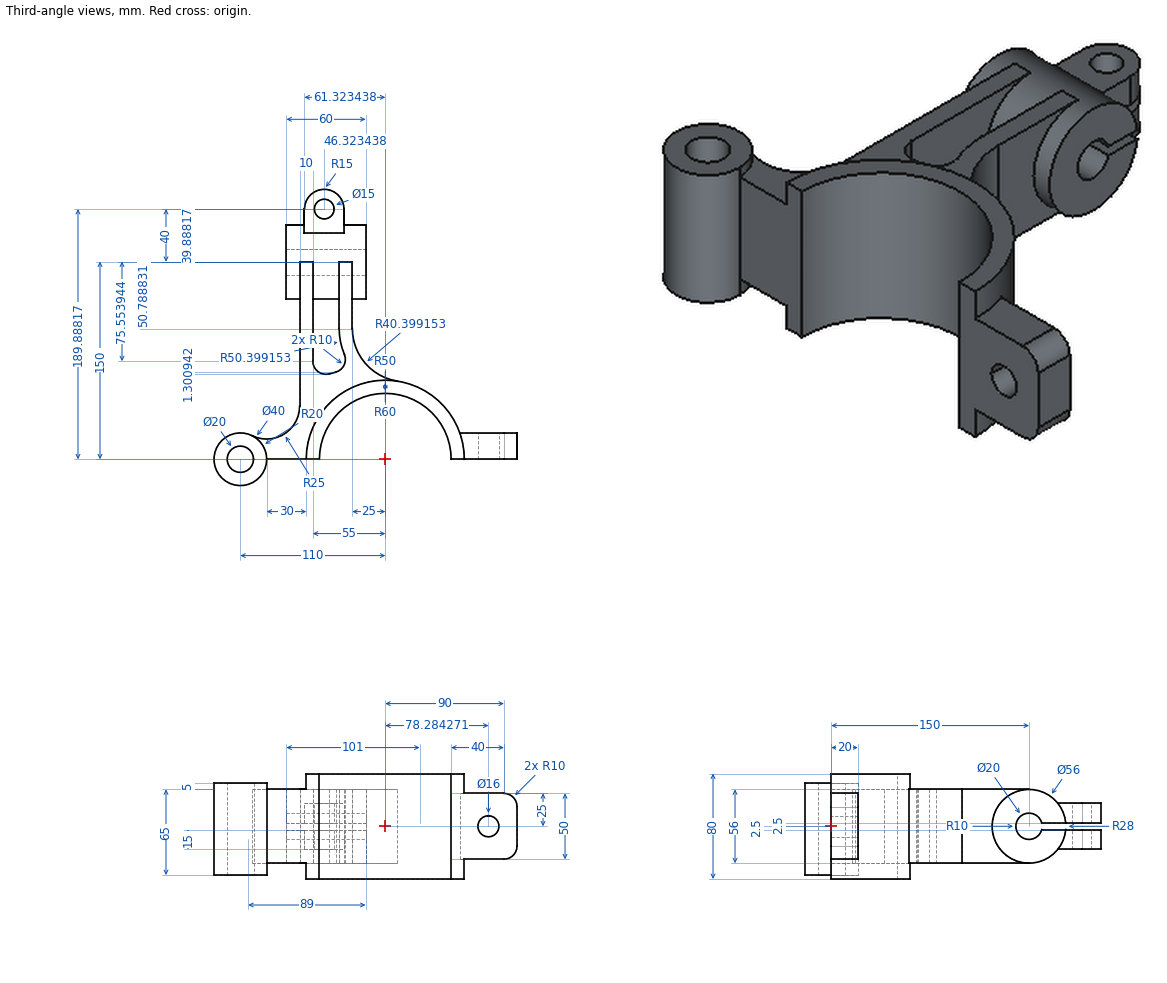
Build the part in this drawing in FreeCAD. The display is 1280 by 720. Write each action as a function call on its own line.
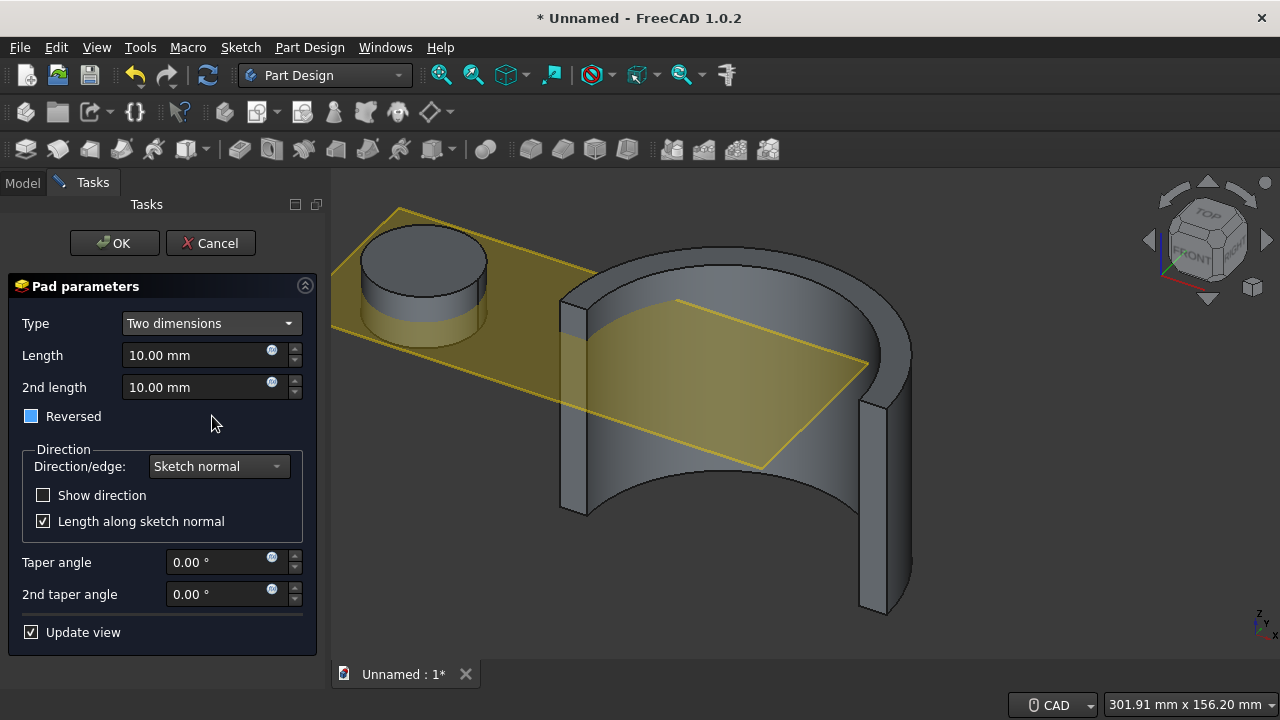
triple_click(204, 355)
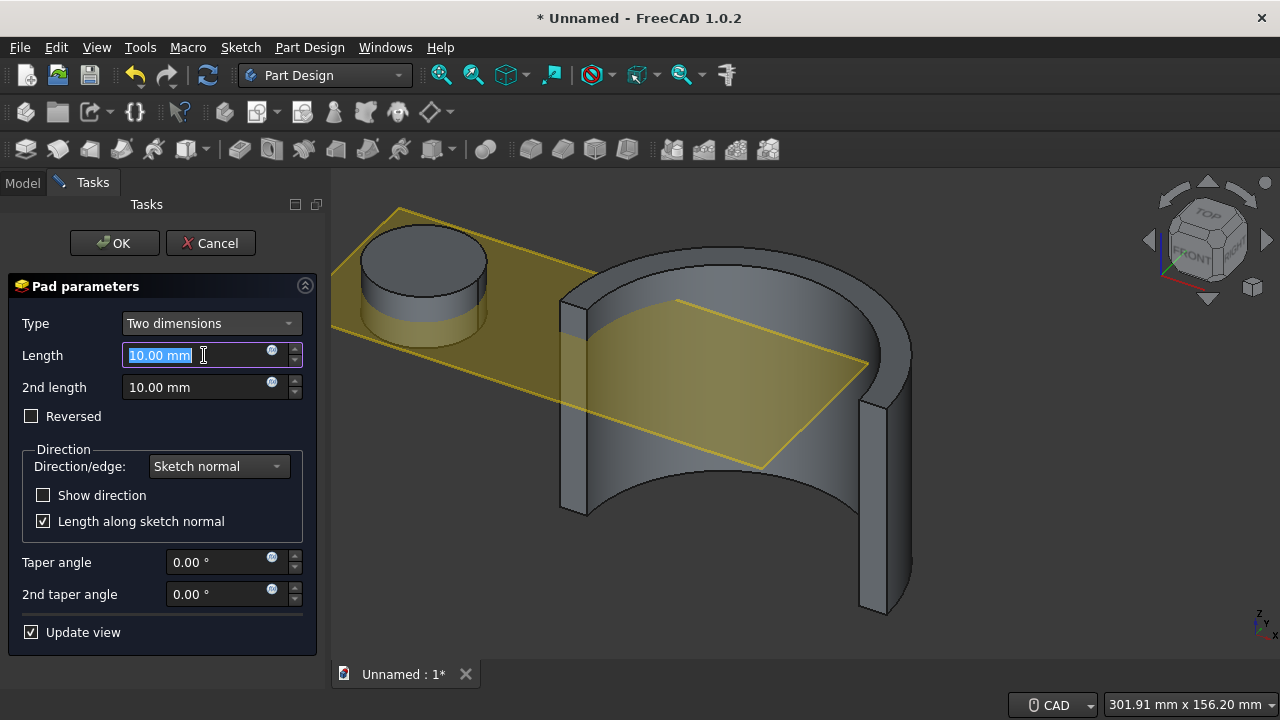
text(5)
key(Tab)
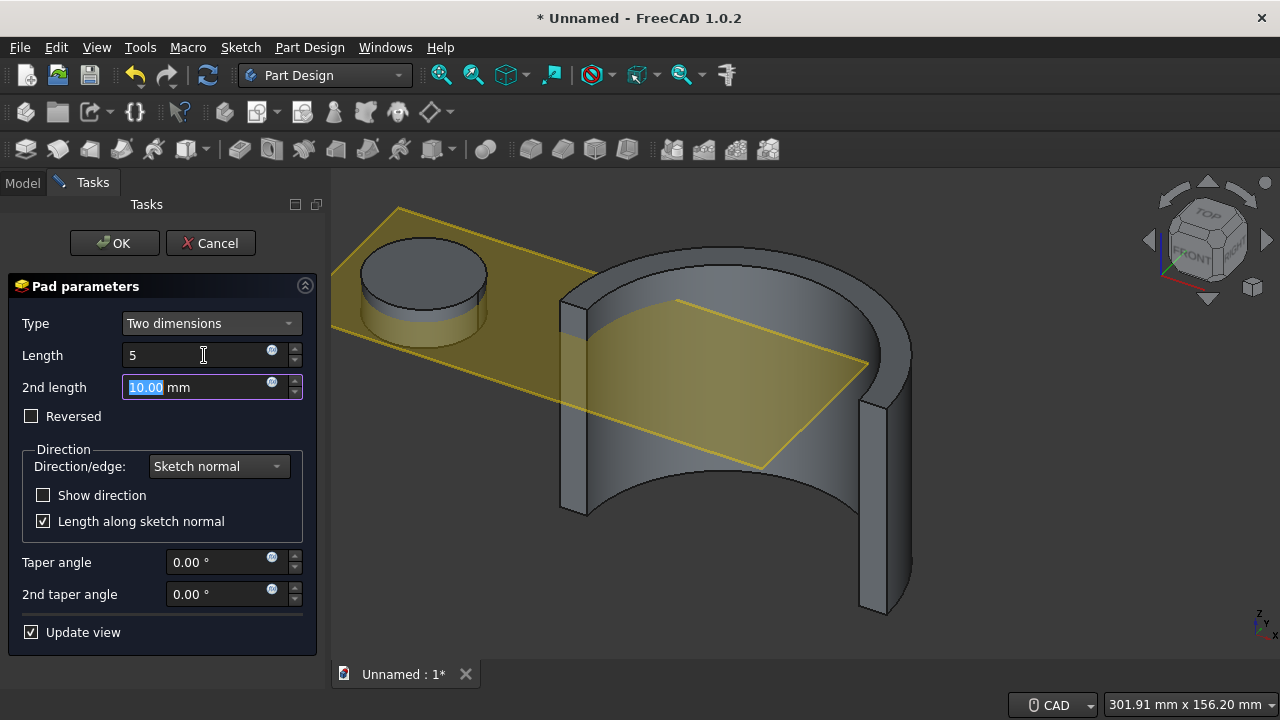
text(65)
key(Tab)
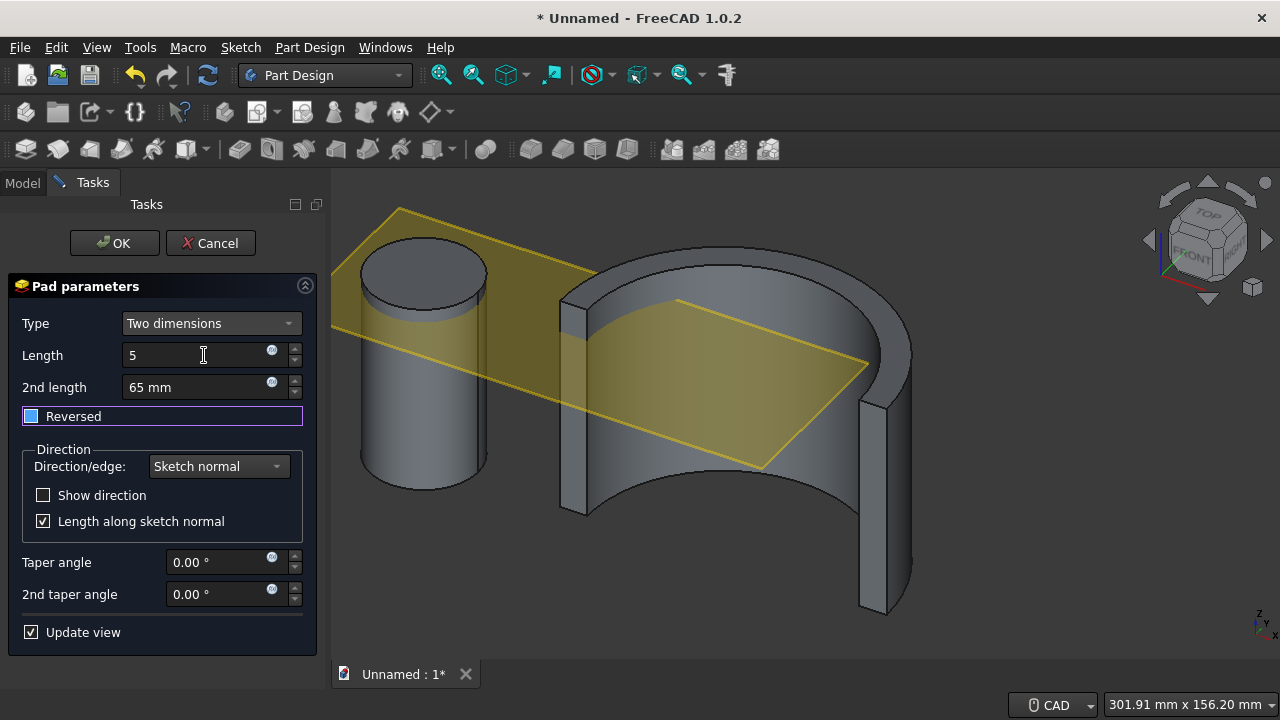
click(115, 243)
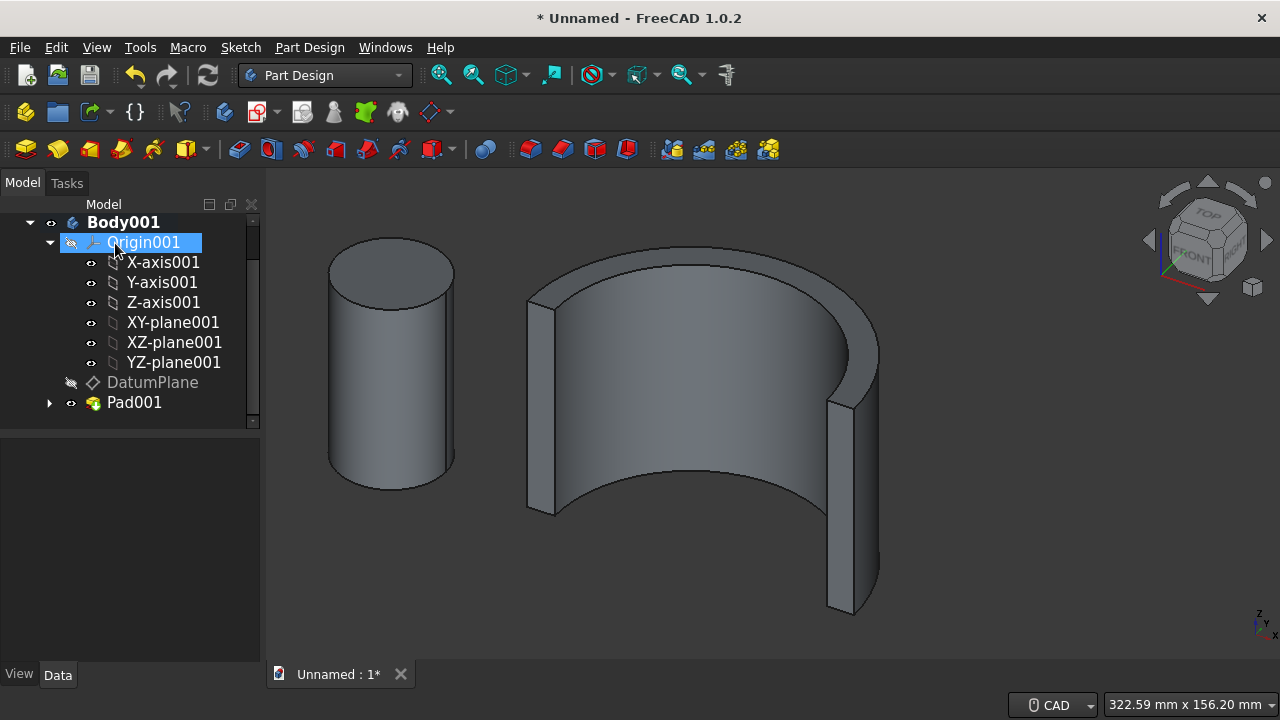
click(226, 112)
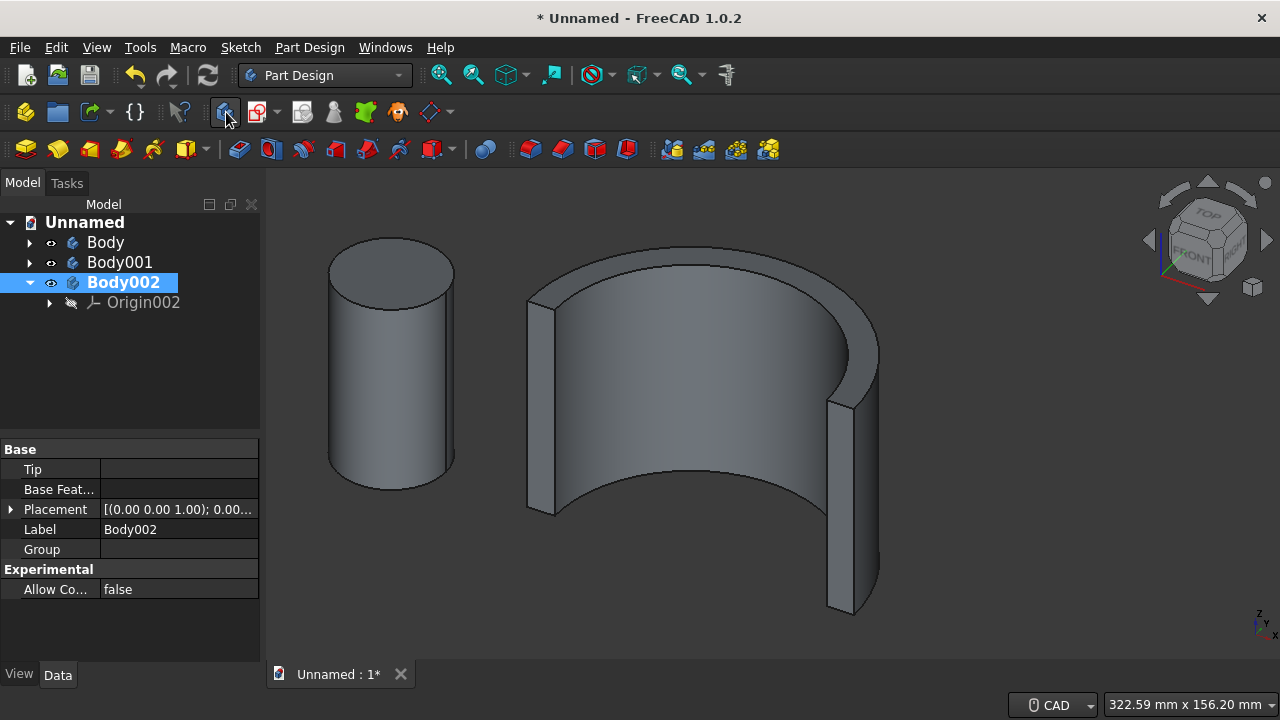
click(50, 303)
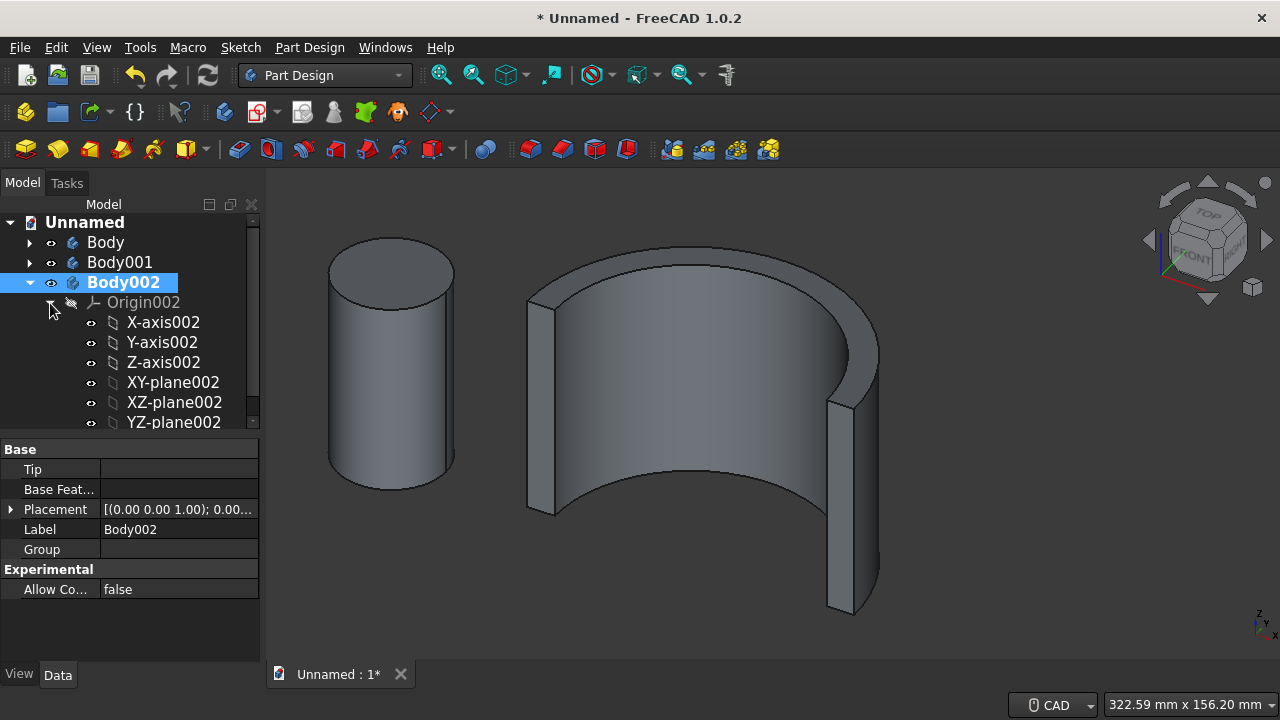
click(136, 423)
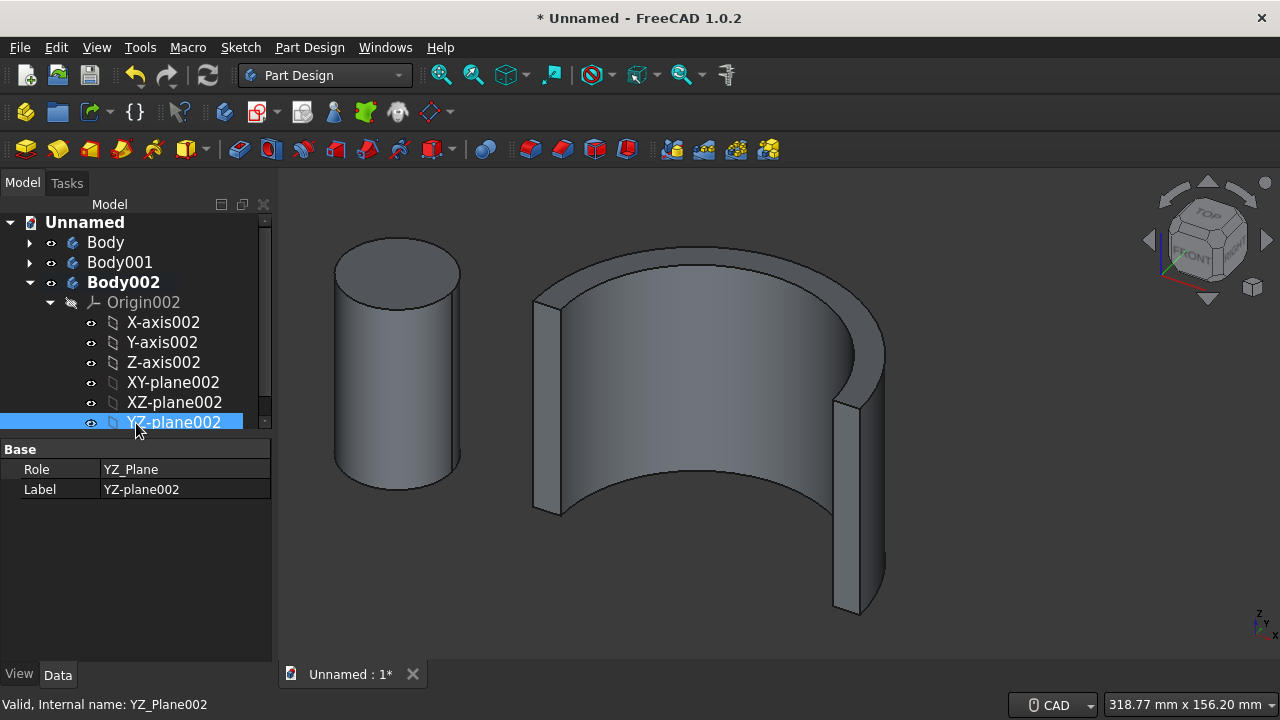
click(430, 112)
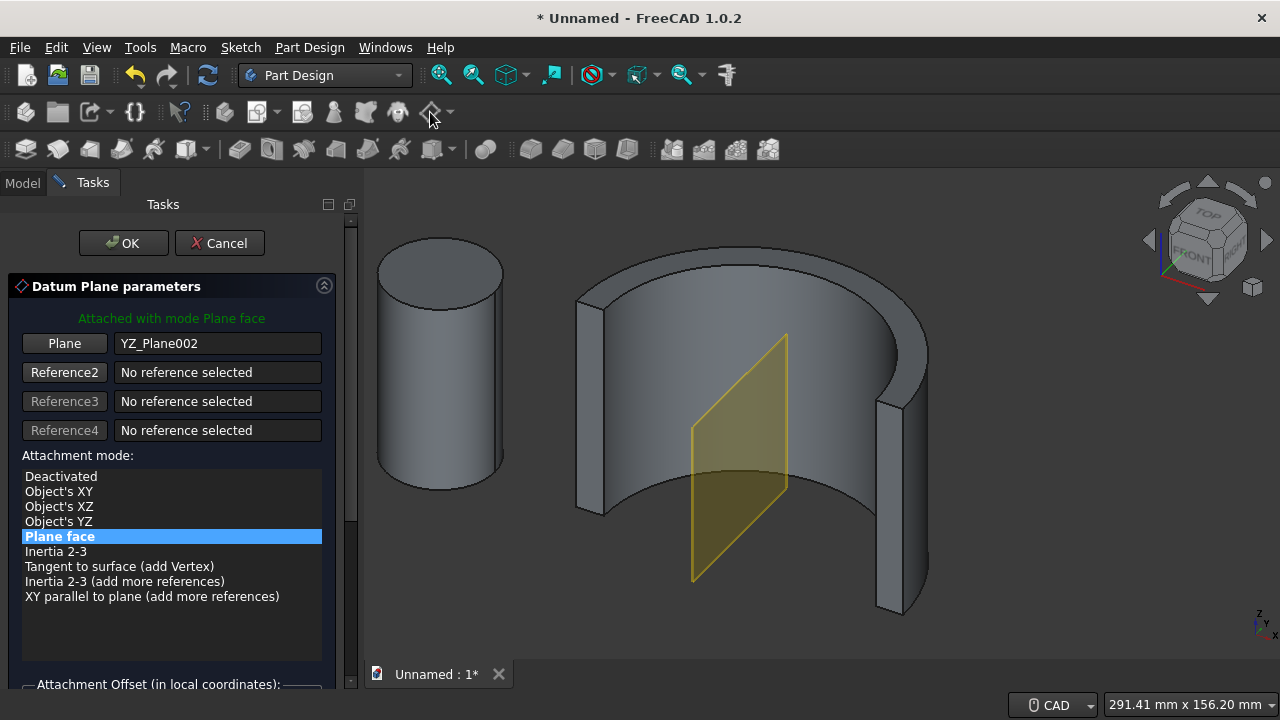
scroll(351, 451, down, 3)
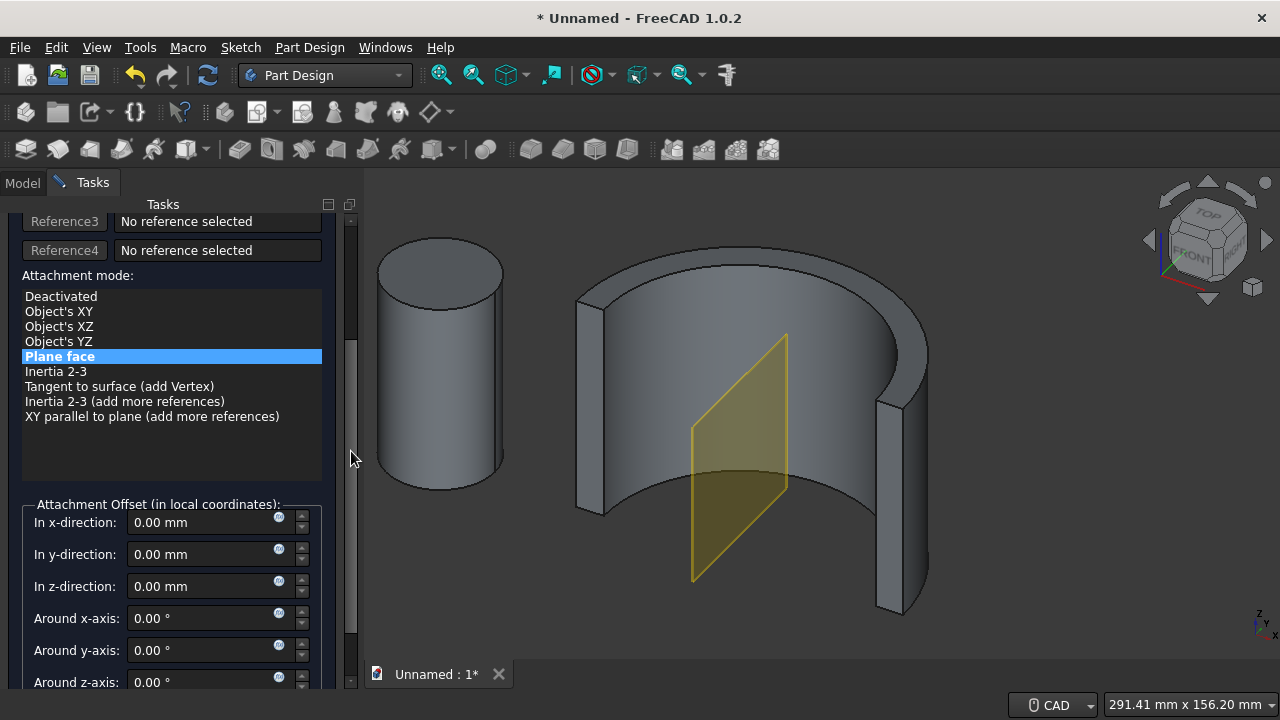
triple_click(210, 586)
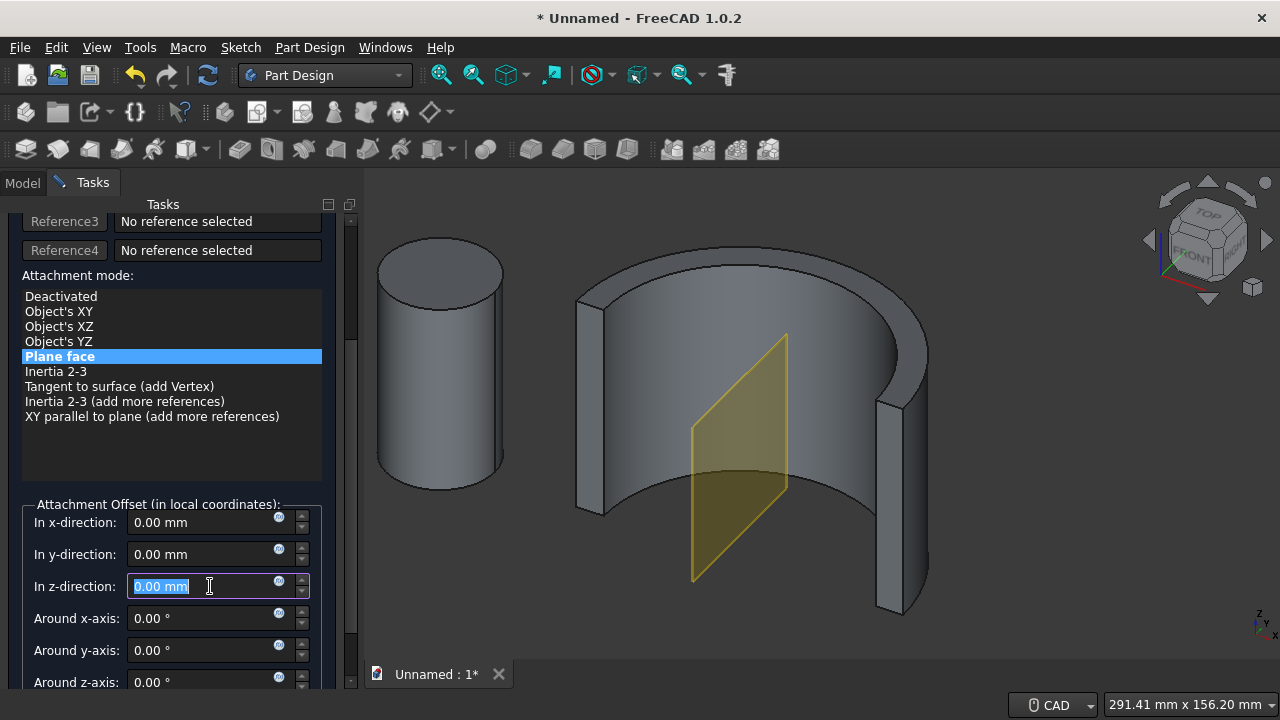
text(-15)
key(Tab)